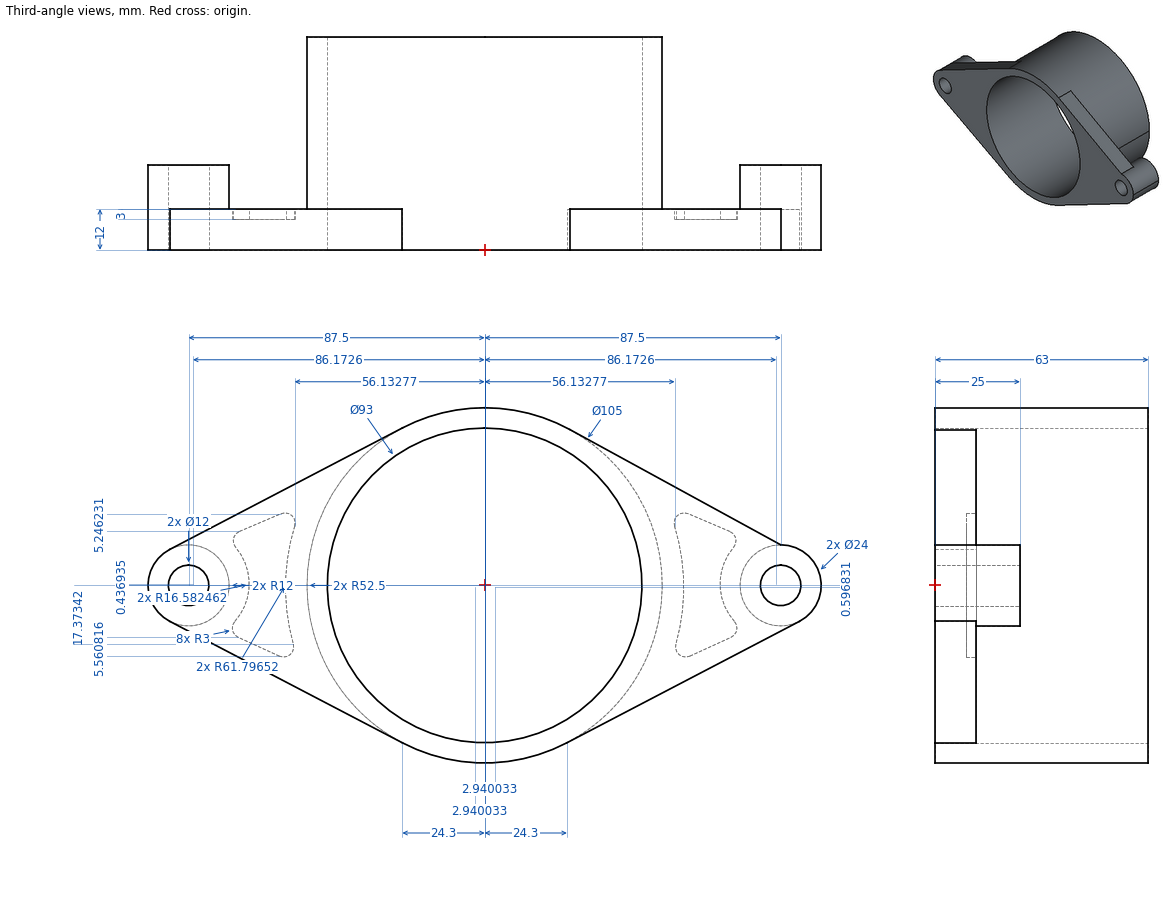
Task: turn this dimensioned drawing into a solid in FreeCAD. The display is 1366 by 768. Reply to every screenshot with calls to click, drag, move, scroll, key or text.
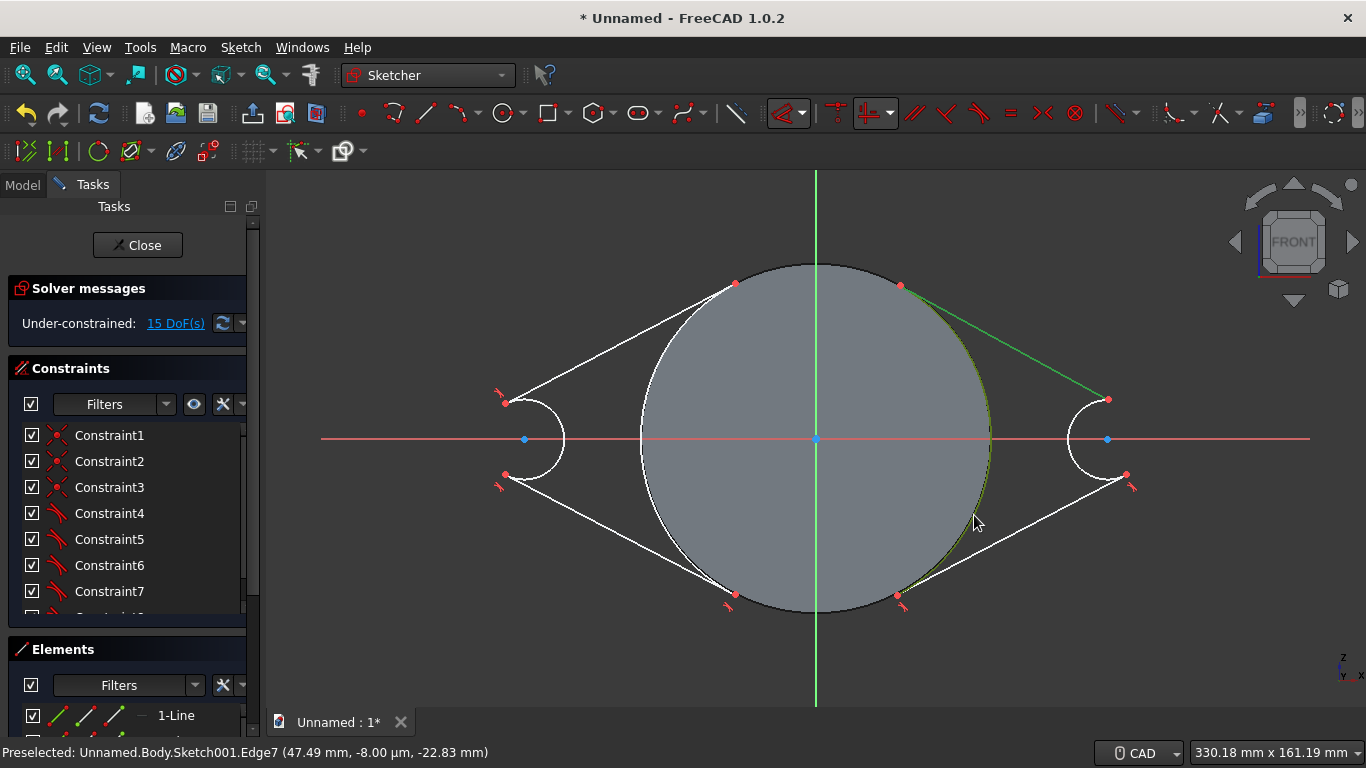
key(t)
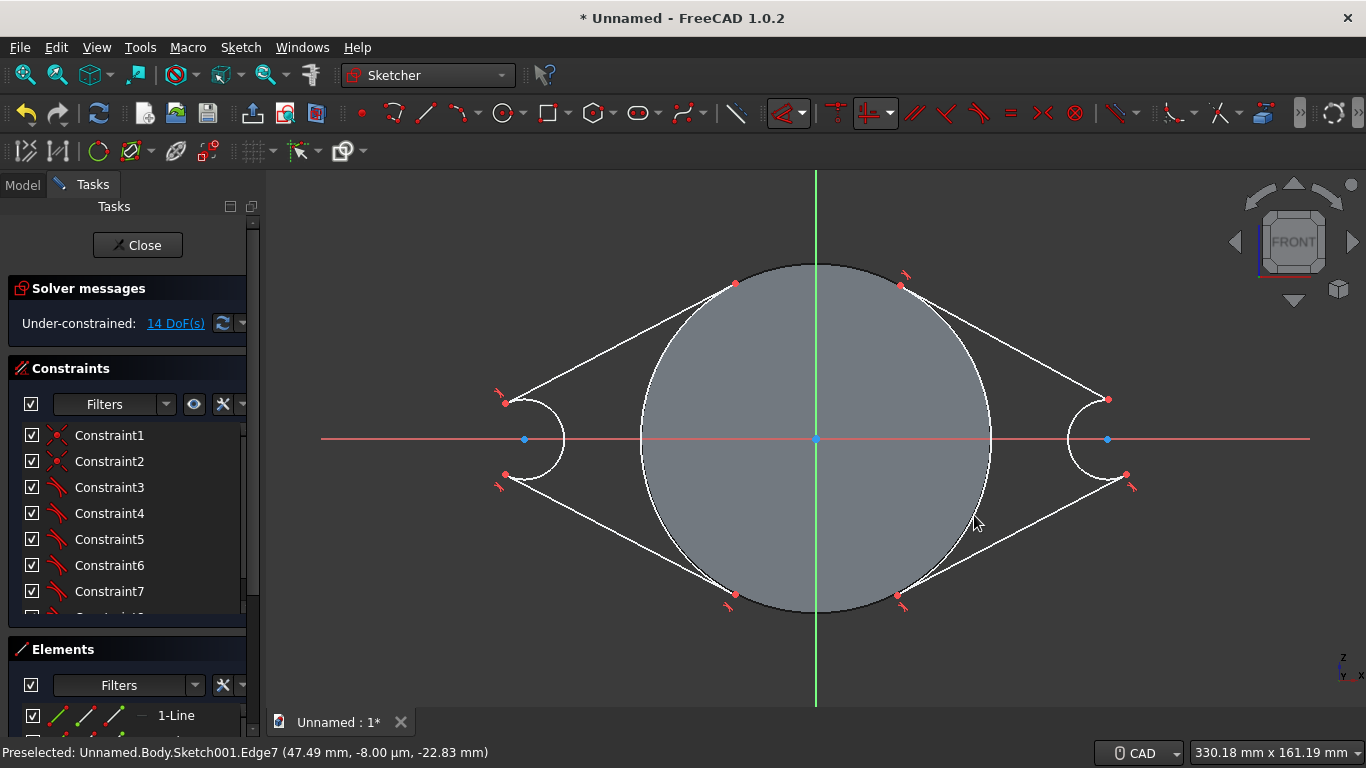
click(657, 365)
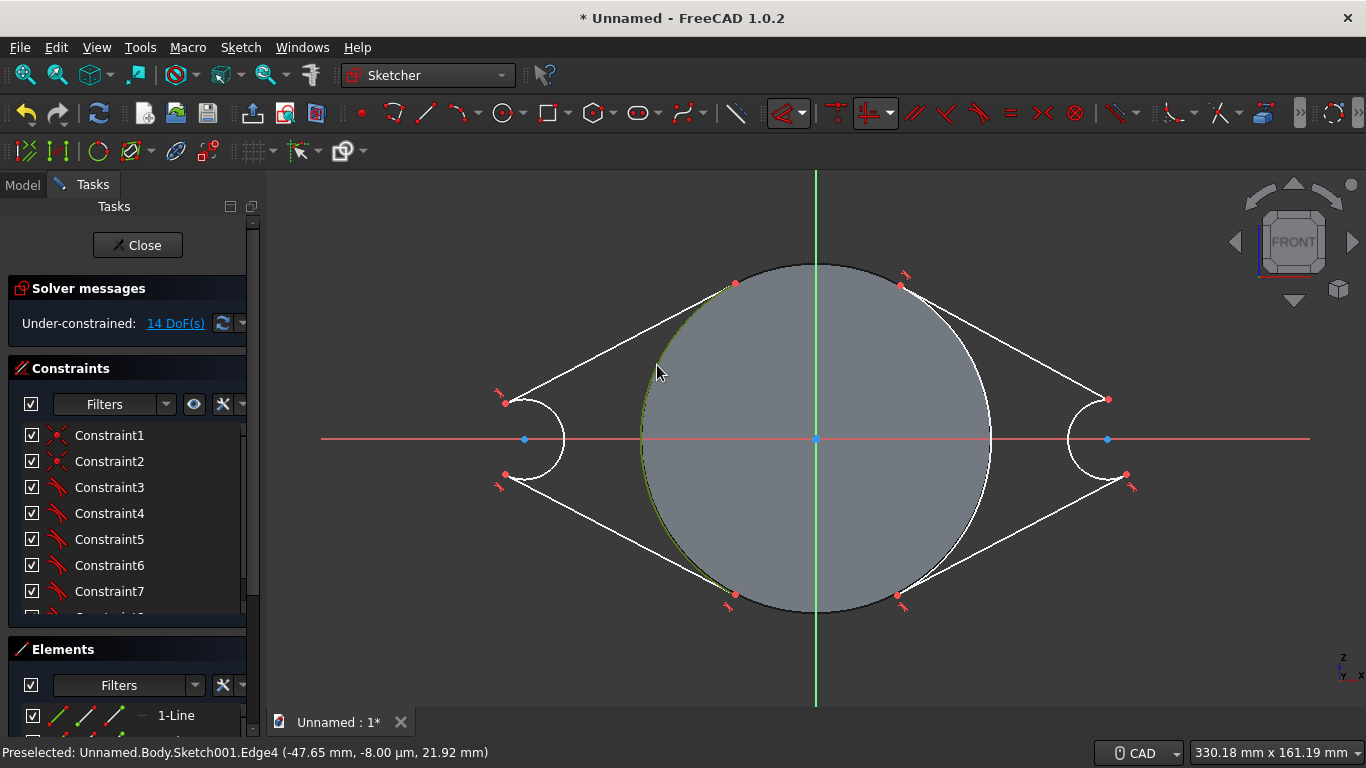
click(974, 515)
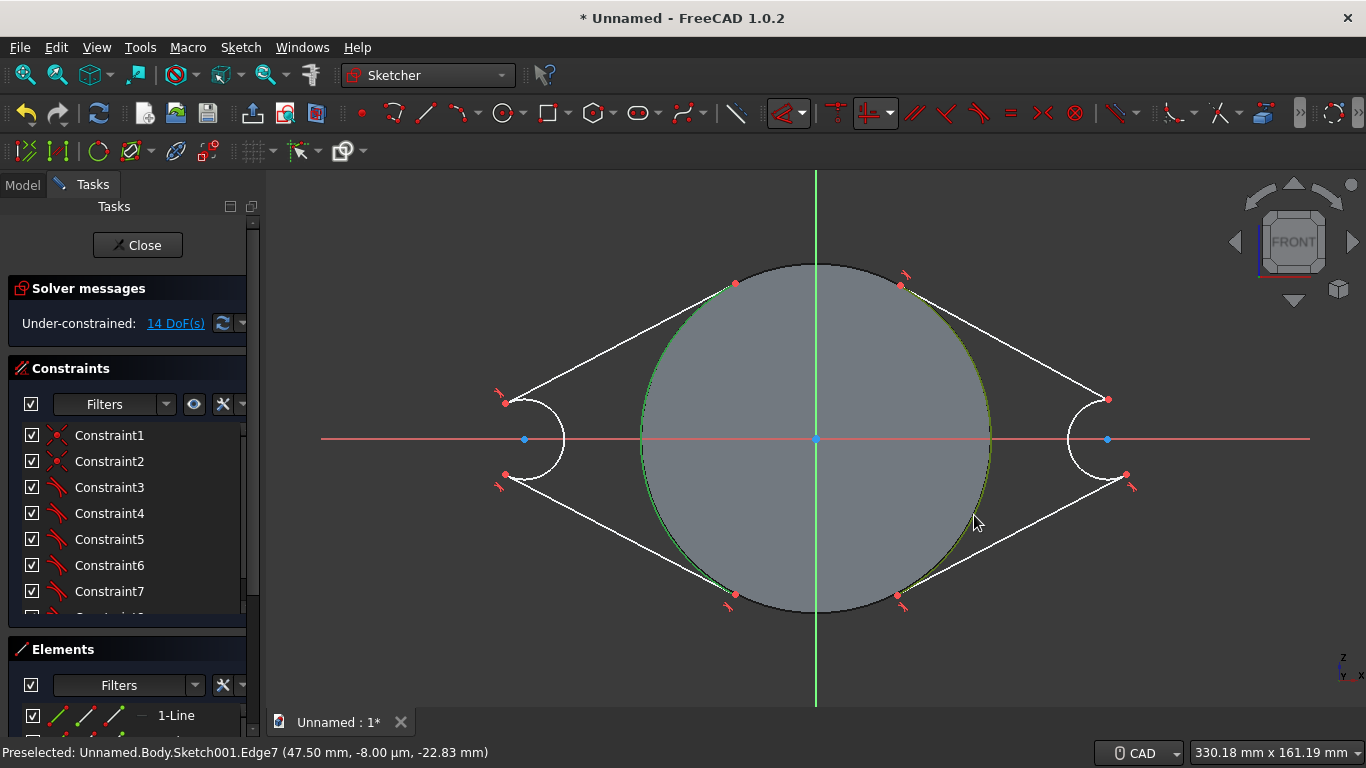
key(c)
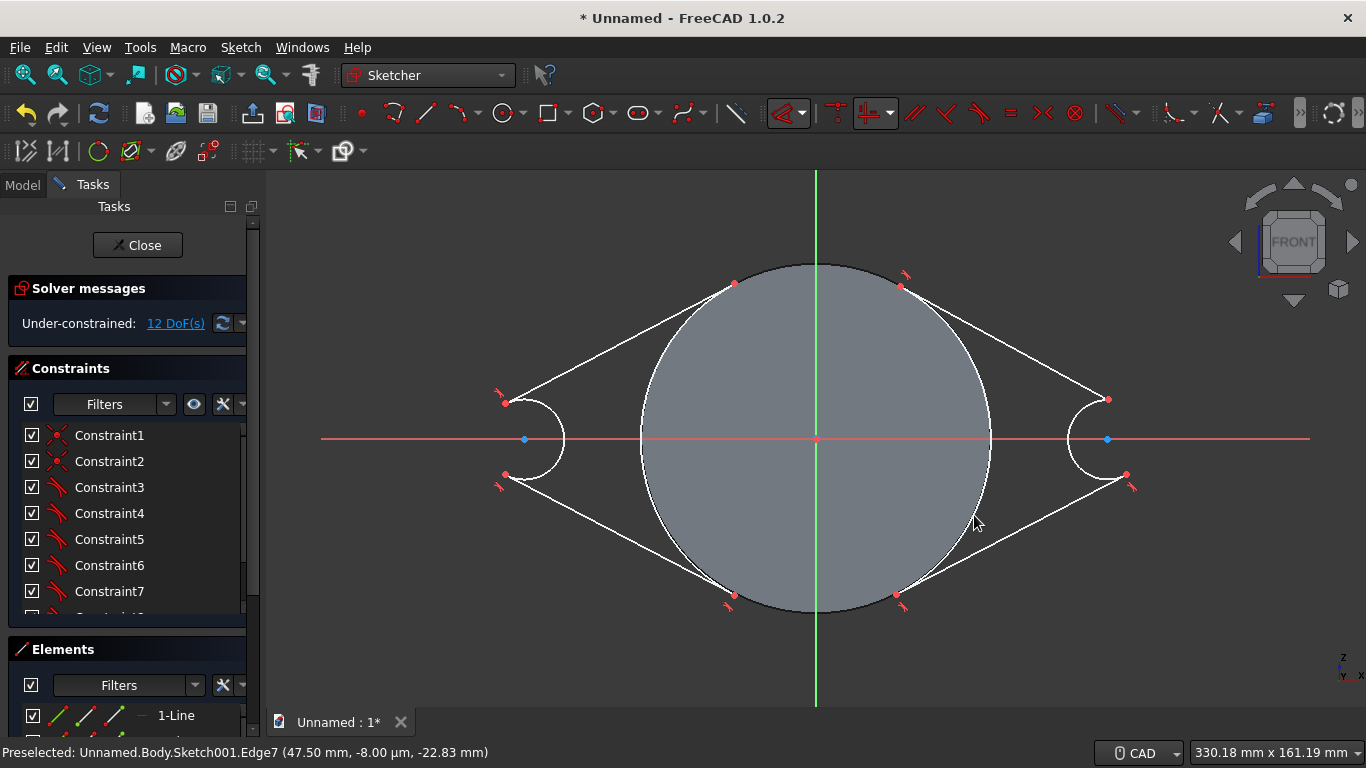
drag(806, 429, 826, 450)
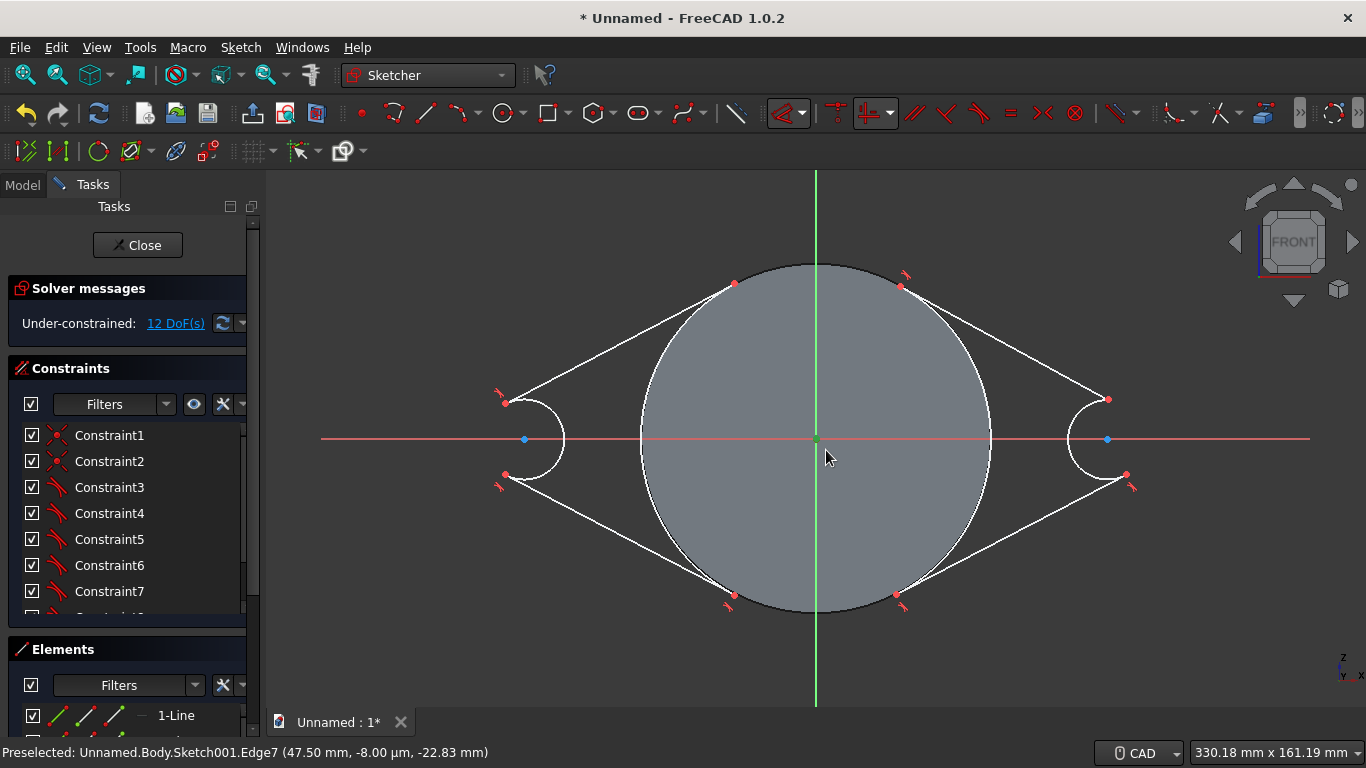
key(c)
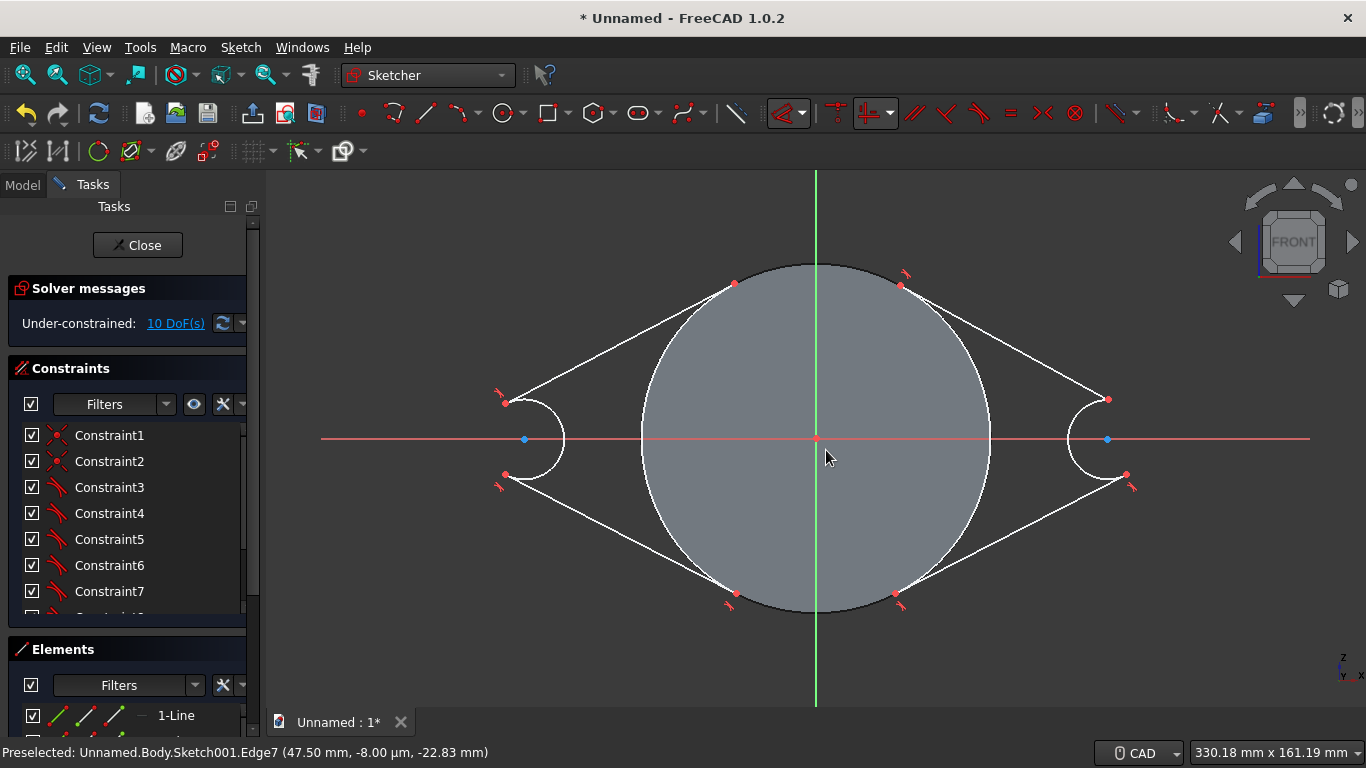
click(658, 365)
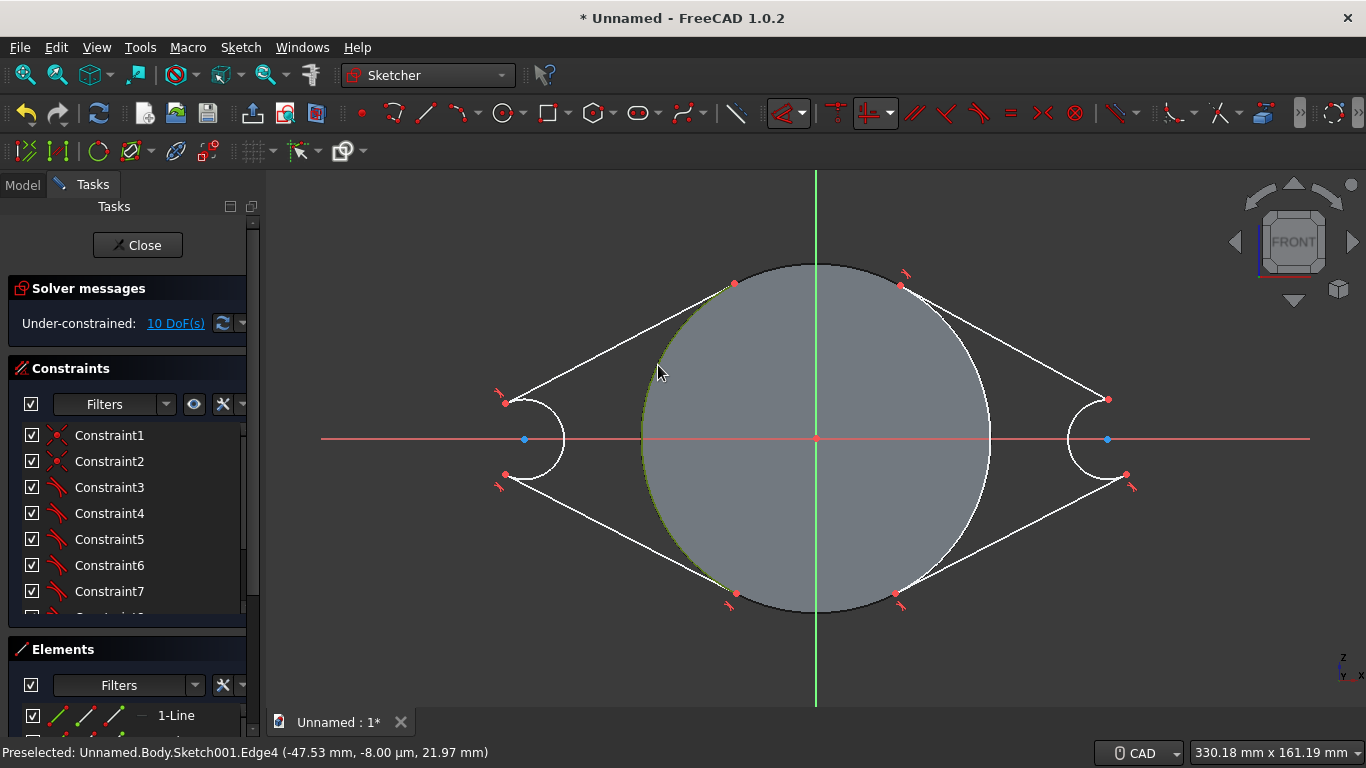
click(973, 514)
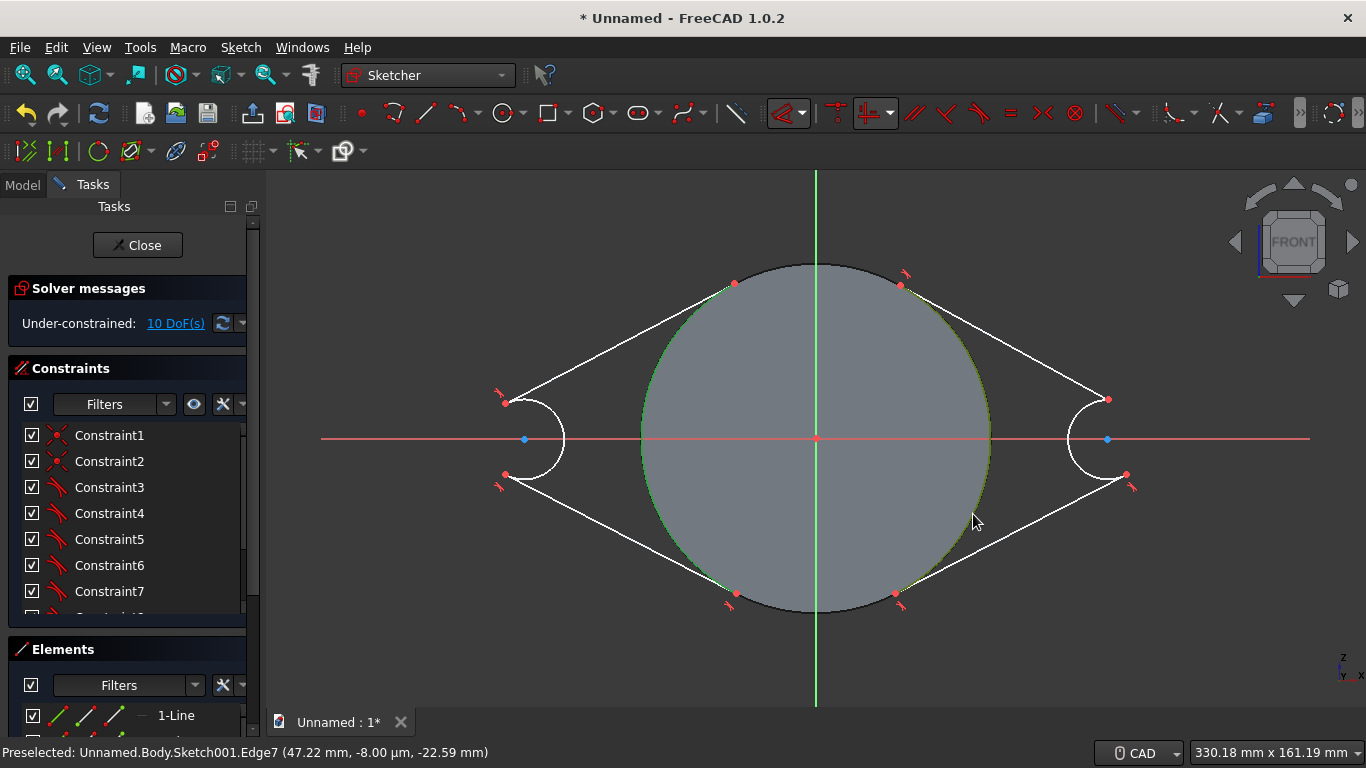
key(e)